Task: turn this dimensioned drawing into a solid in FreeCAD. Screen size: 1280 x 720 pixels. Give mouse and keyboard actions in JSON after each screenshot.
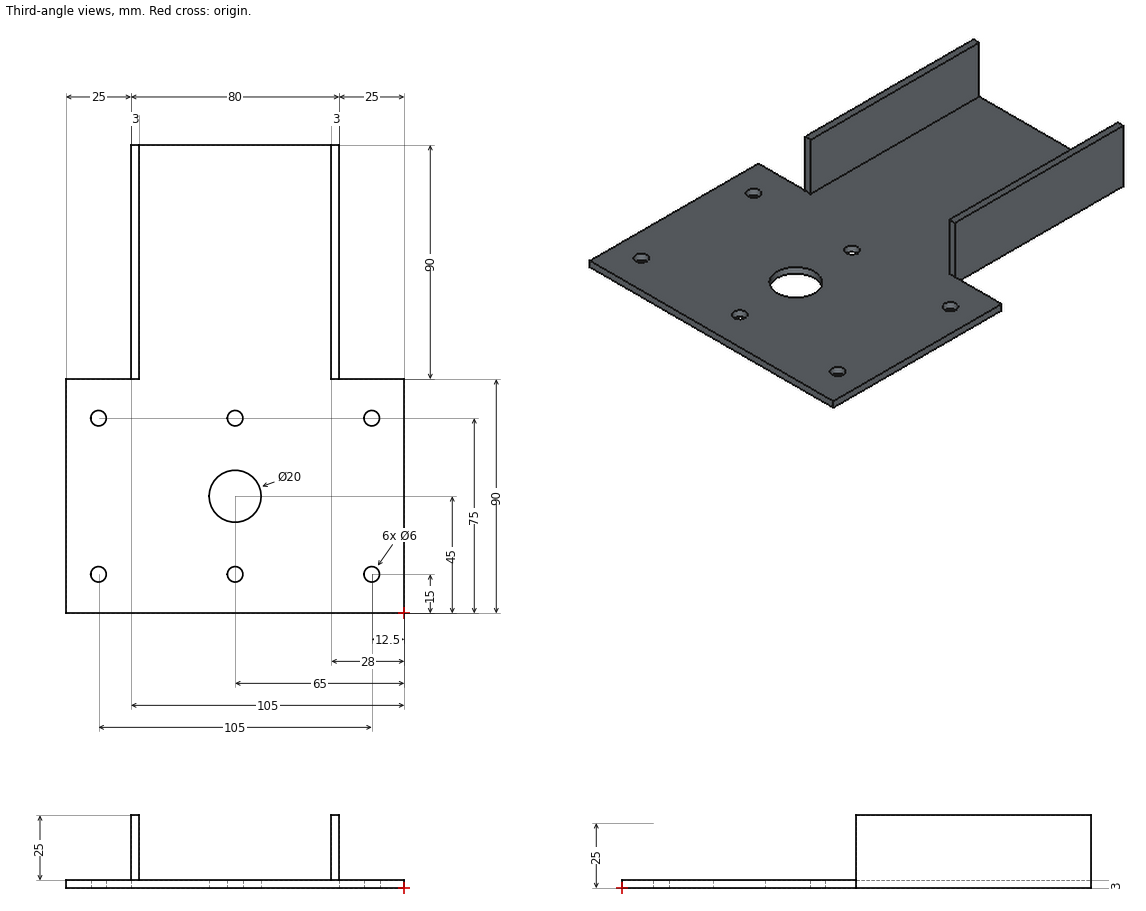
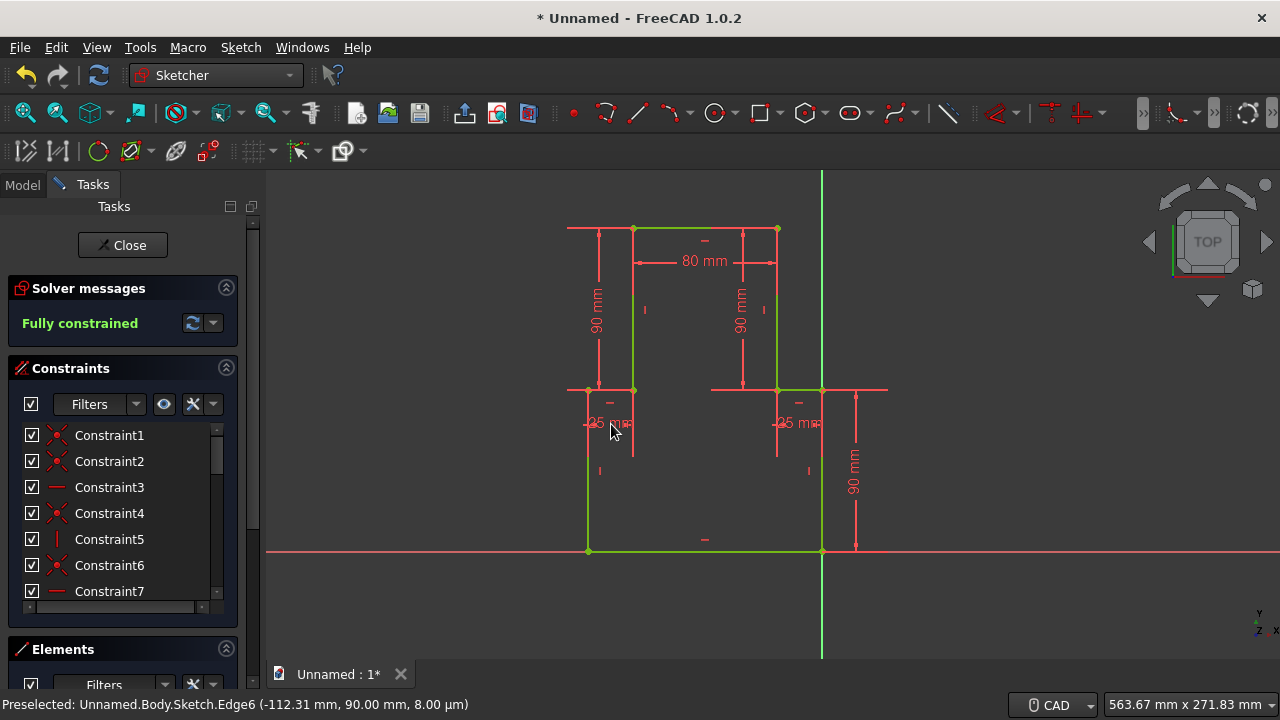
{"action": "left_click", "coordinate": [123, 245]}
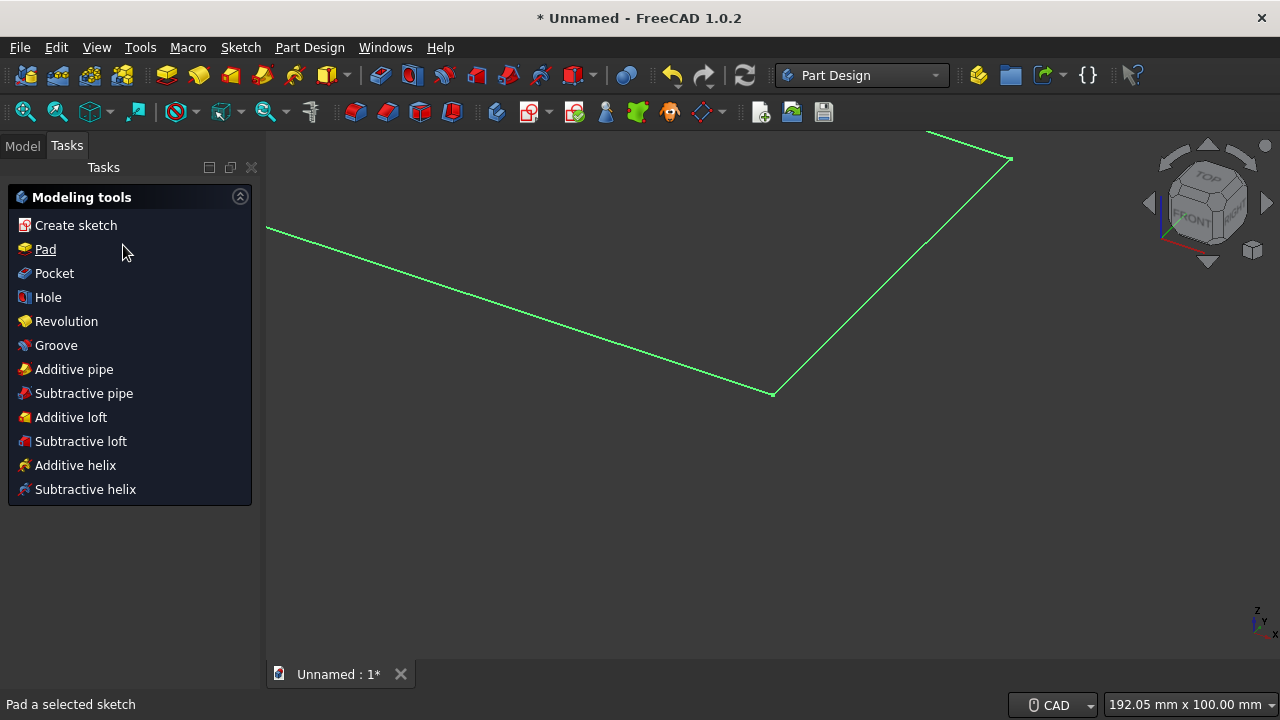
{"action": "left_click", "coordinate": [168, 76]}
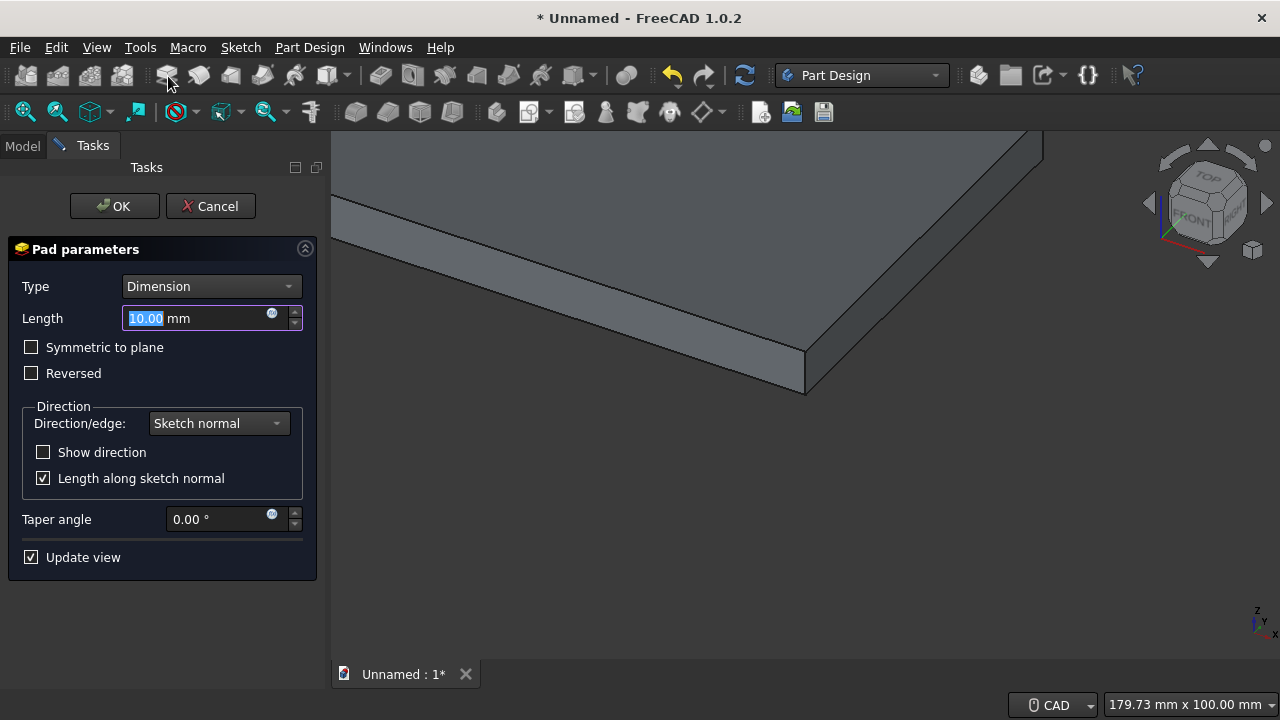
{"action": "type", "text": "3"}
{"action": "key", "text": "Tab"}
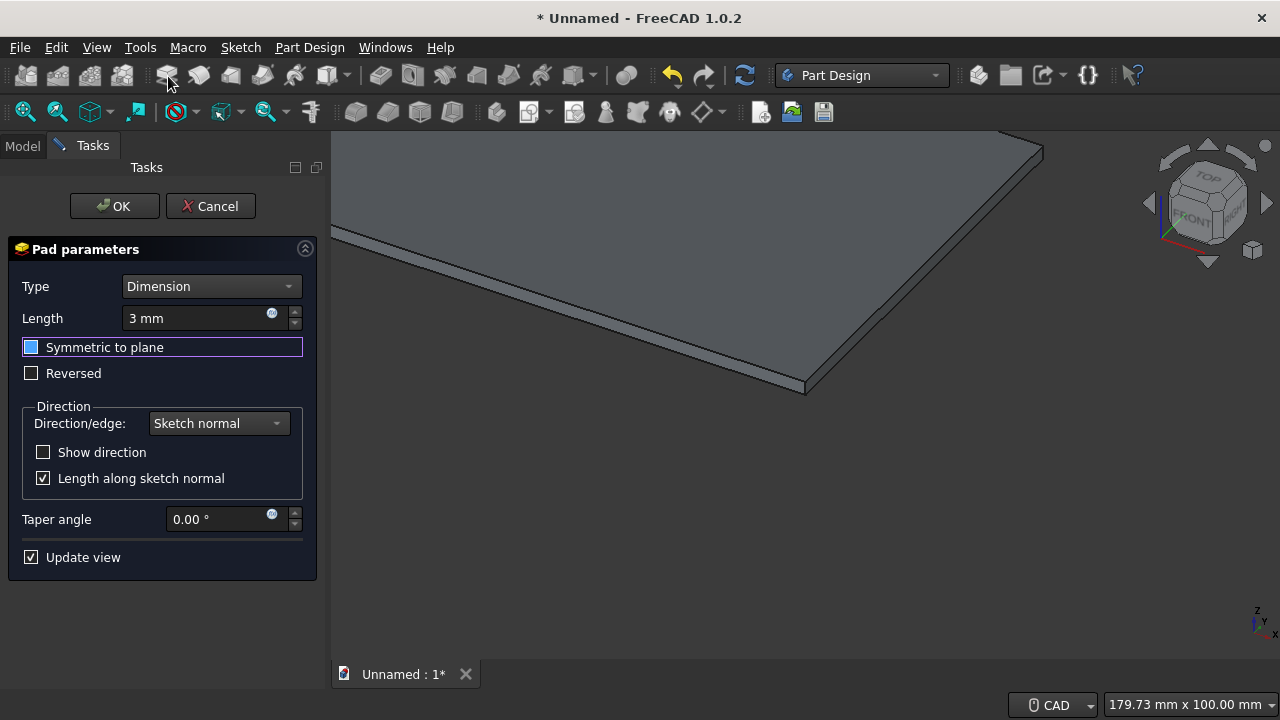
{"action": "left_click", "coordinate": [115, 206]}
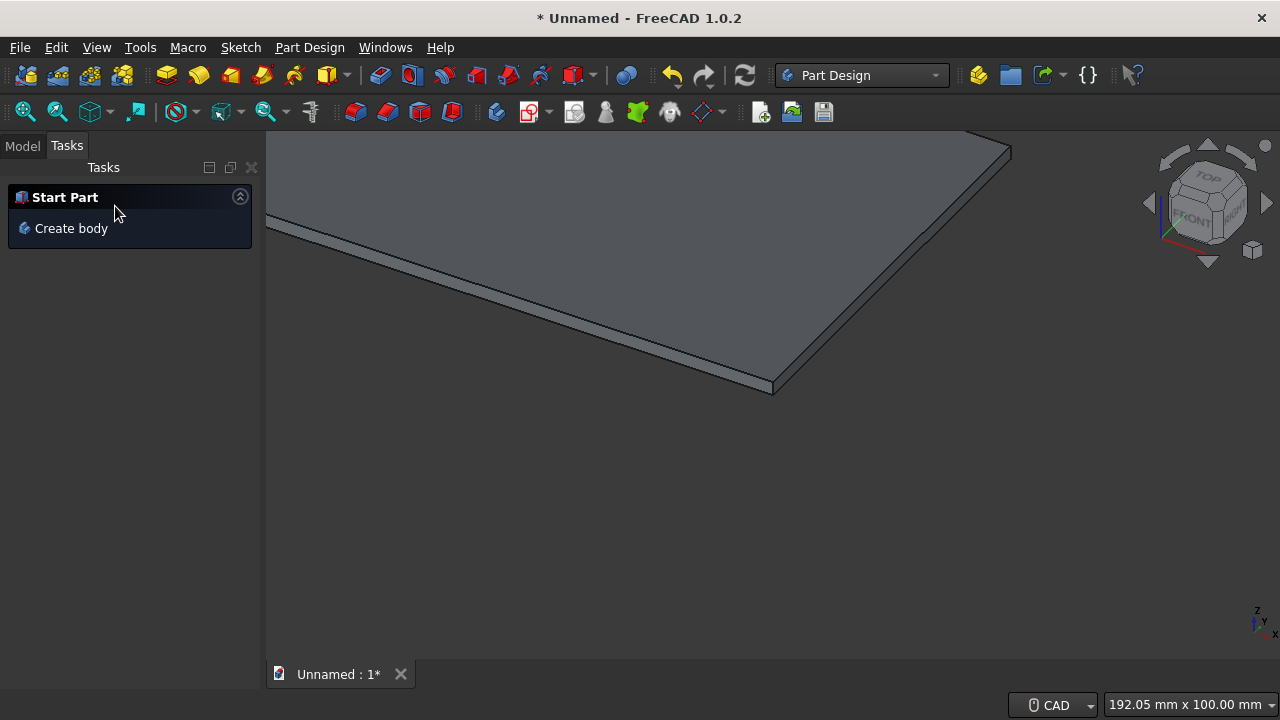
{"action": "left_click", "coordinate": [26, 112]}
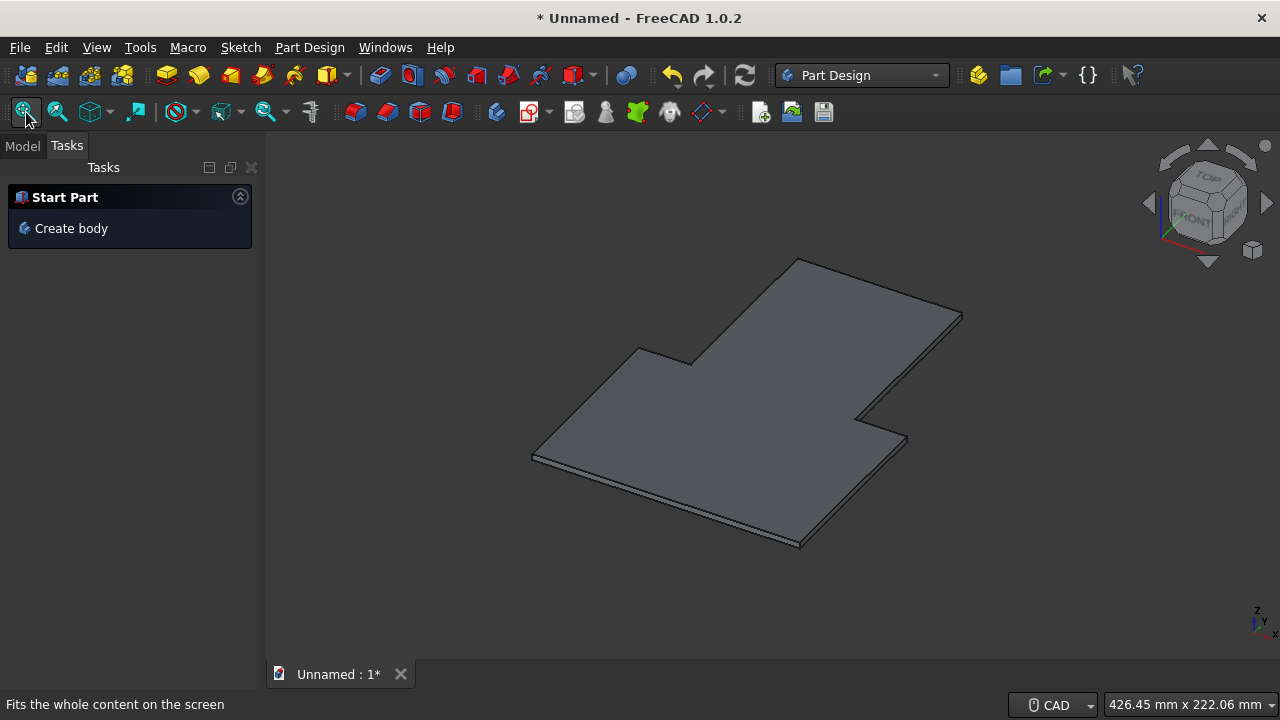
{"action": "left_click", "coordinate": [742, 421]}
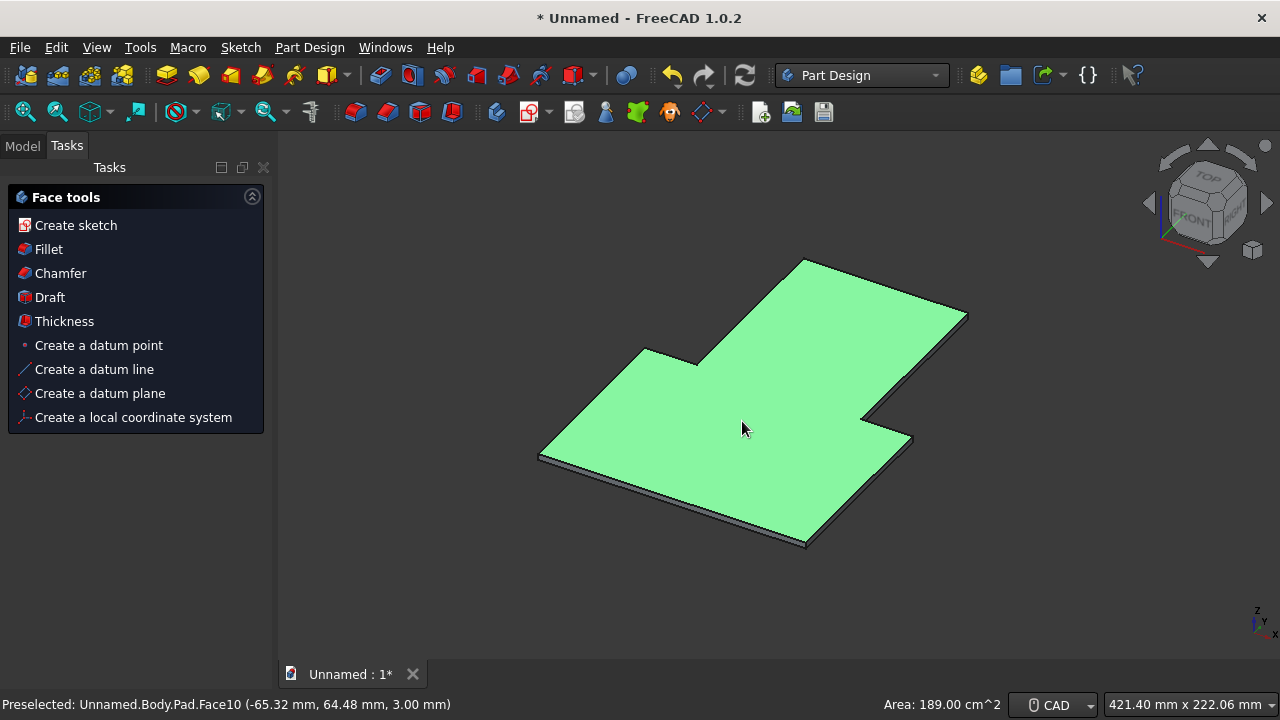
{"action": "left_click", "coordinate": [530, 112]}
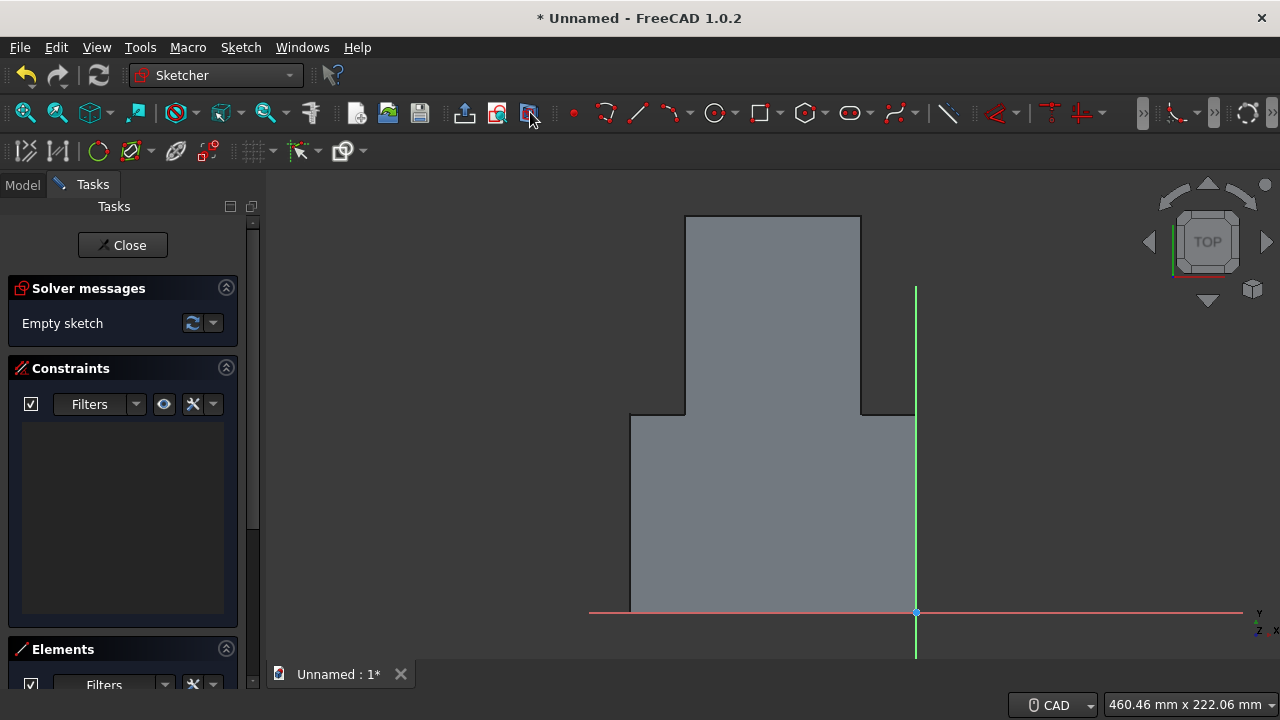
{"action": "scroll", "coordinate": [294, 415], "scroll_direction": "down", "scroll_amount": 1}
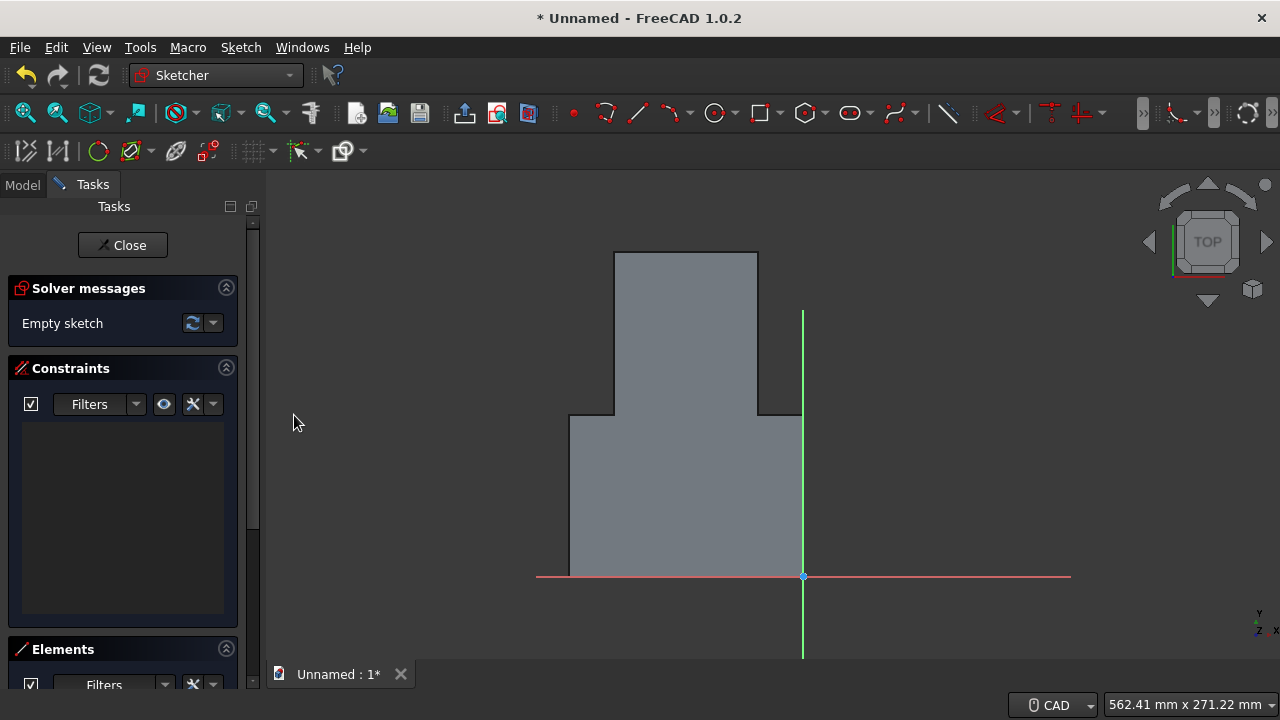
{"action": "left_click", "coordinate": [760, 114]}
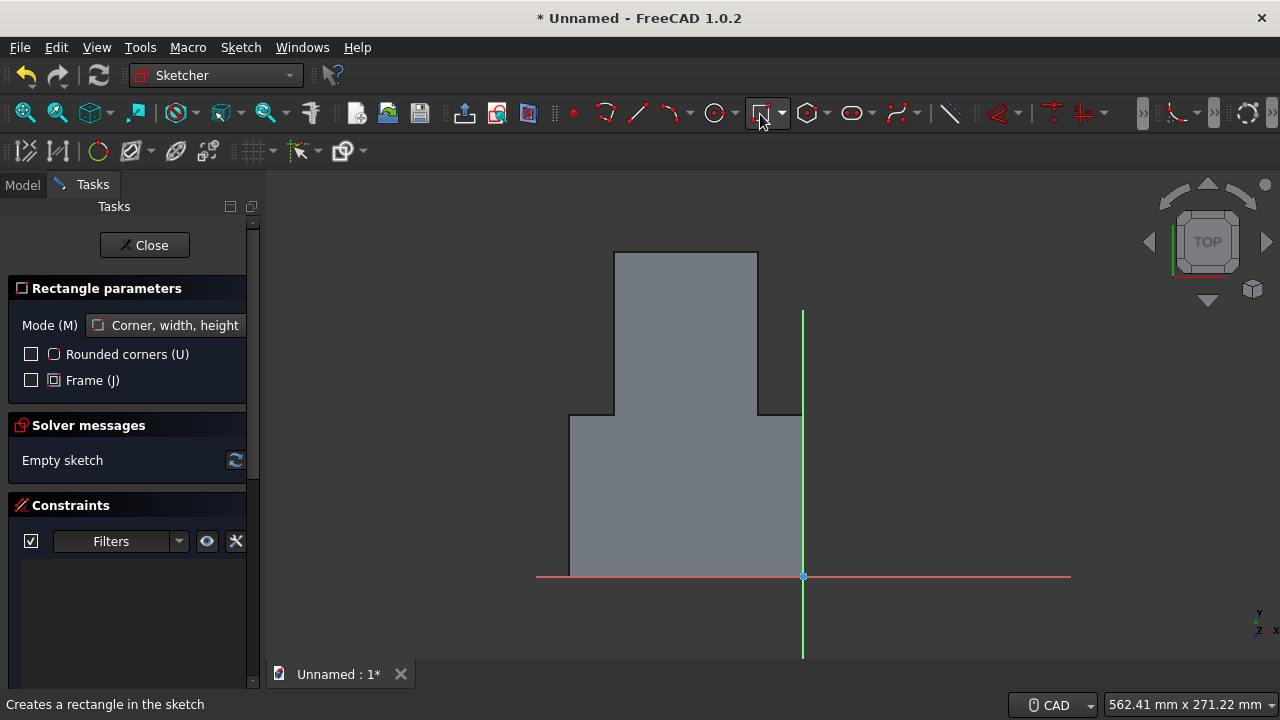
{"action": "scroll", "coordinate": [614, 252], "scroll_direction": "up", "scroll_amount": 6}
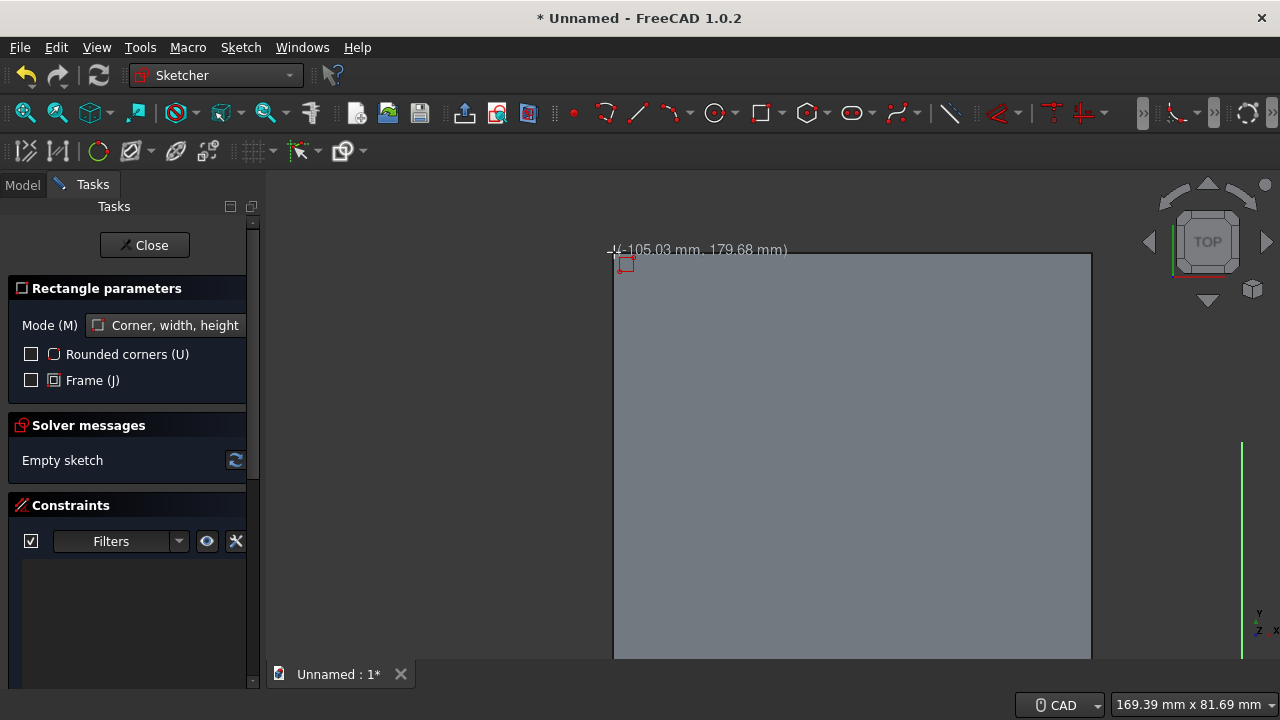
{"action": "left_click", "coordinate": [613, 253]}